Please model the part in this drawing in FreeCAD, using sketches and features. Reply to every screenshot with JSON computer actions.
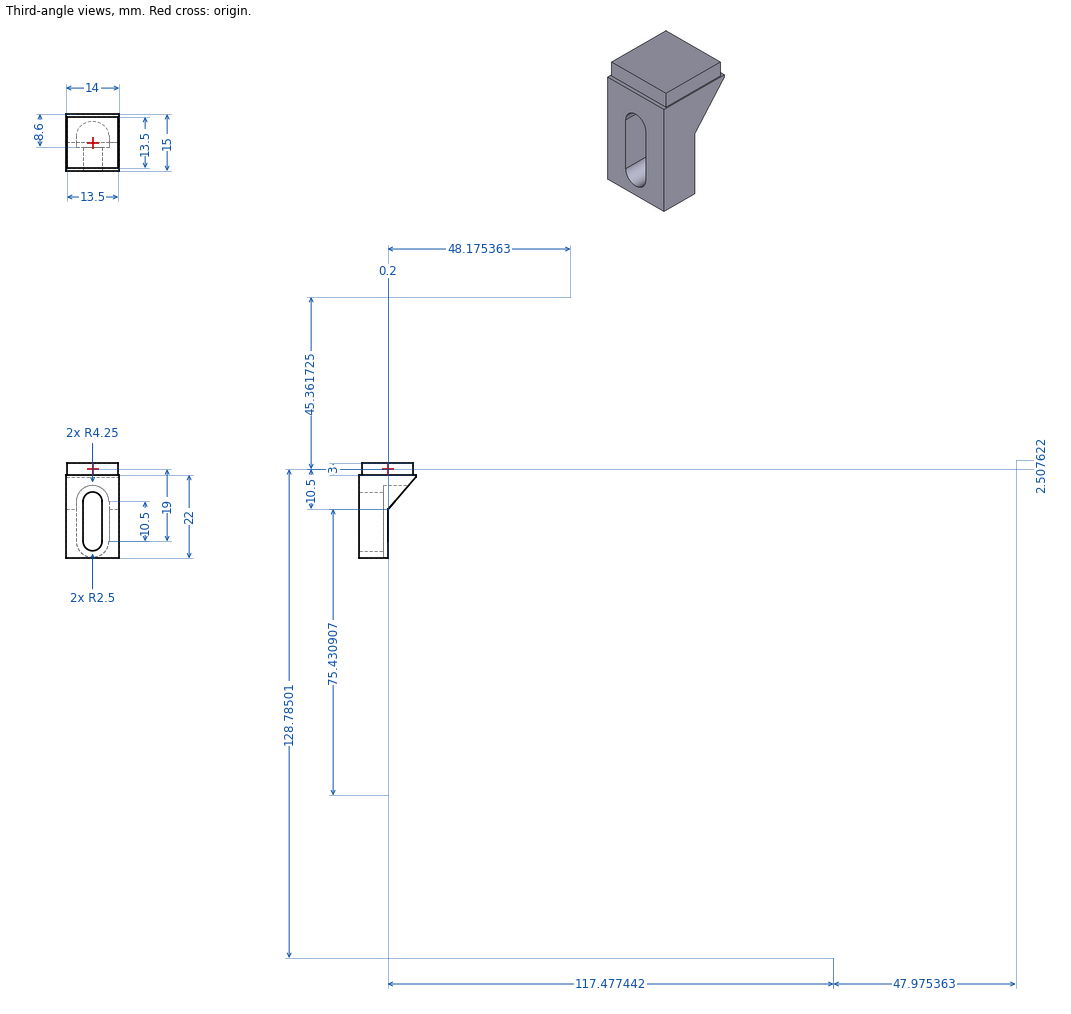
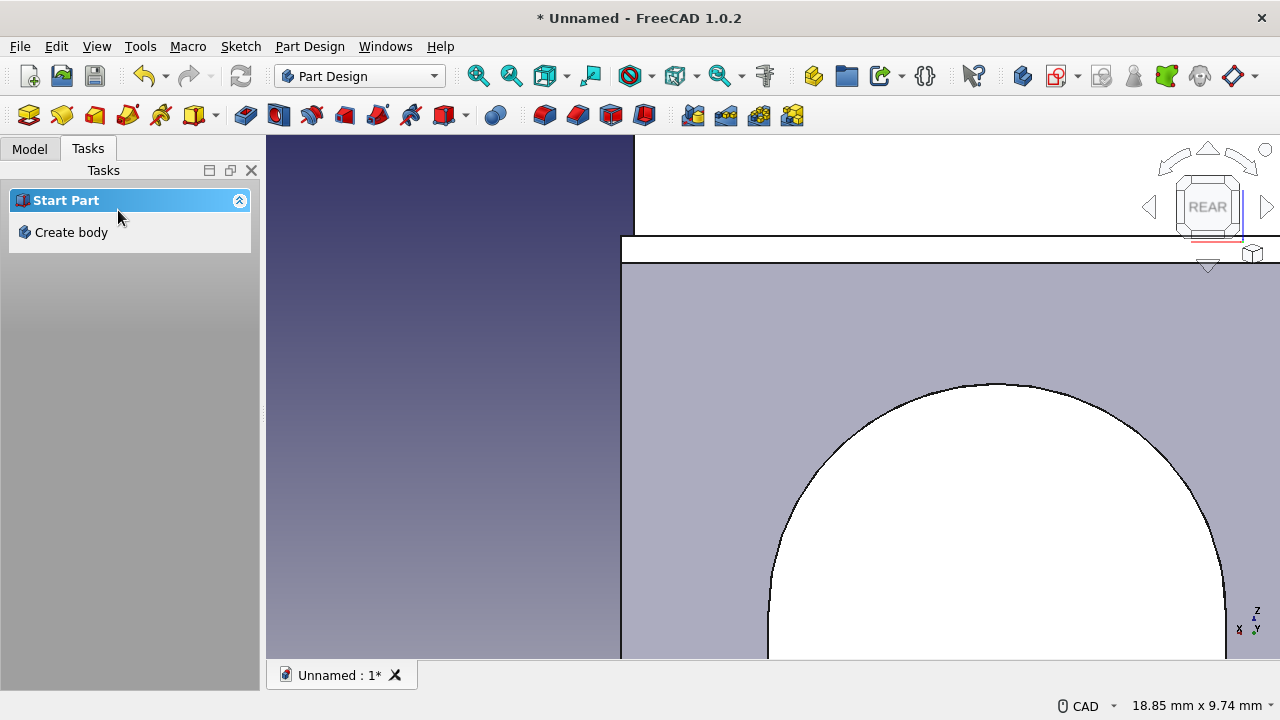
{"action": "key", "text": "v f"}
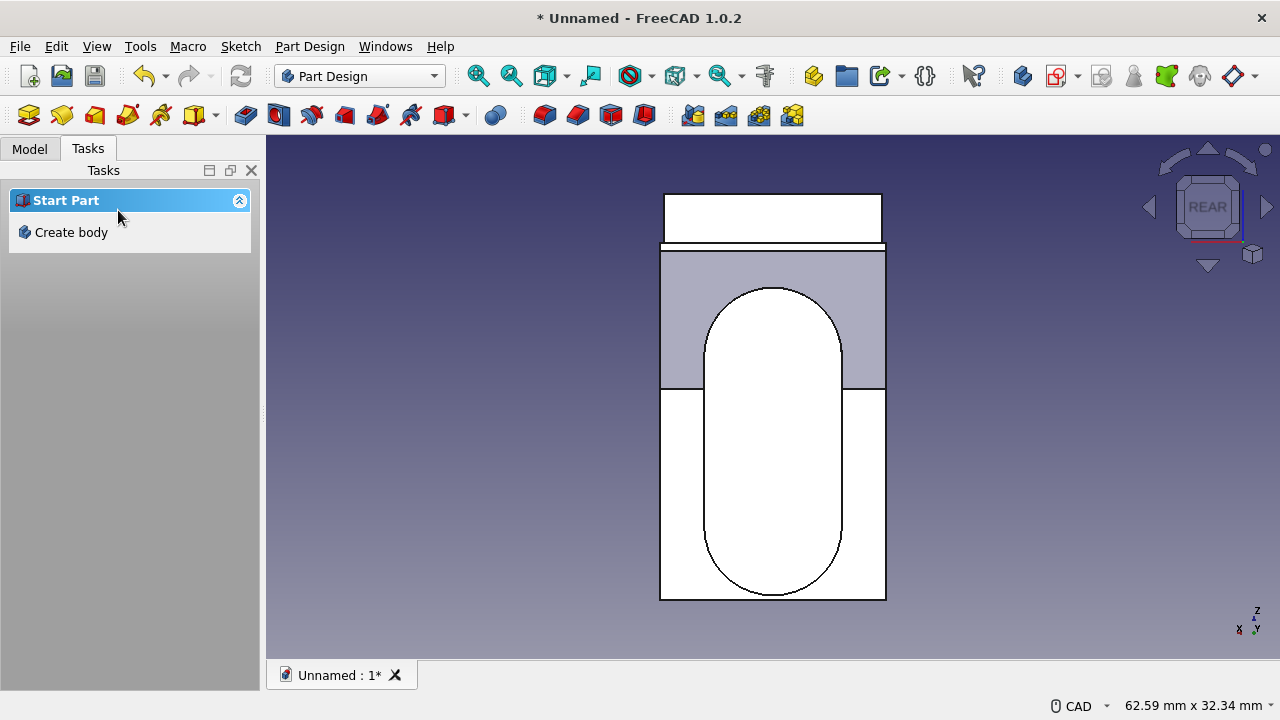
{"action": "left_click", "coordinate": [676, 433]}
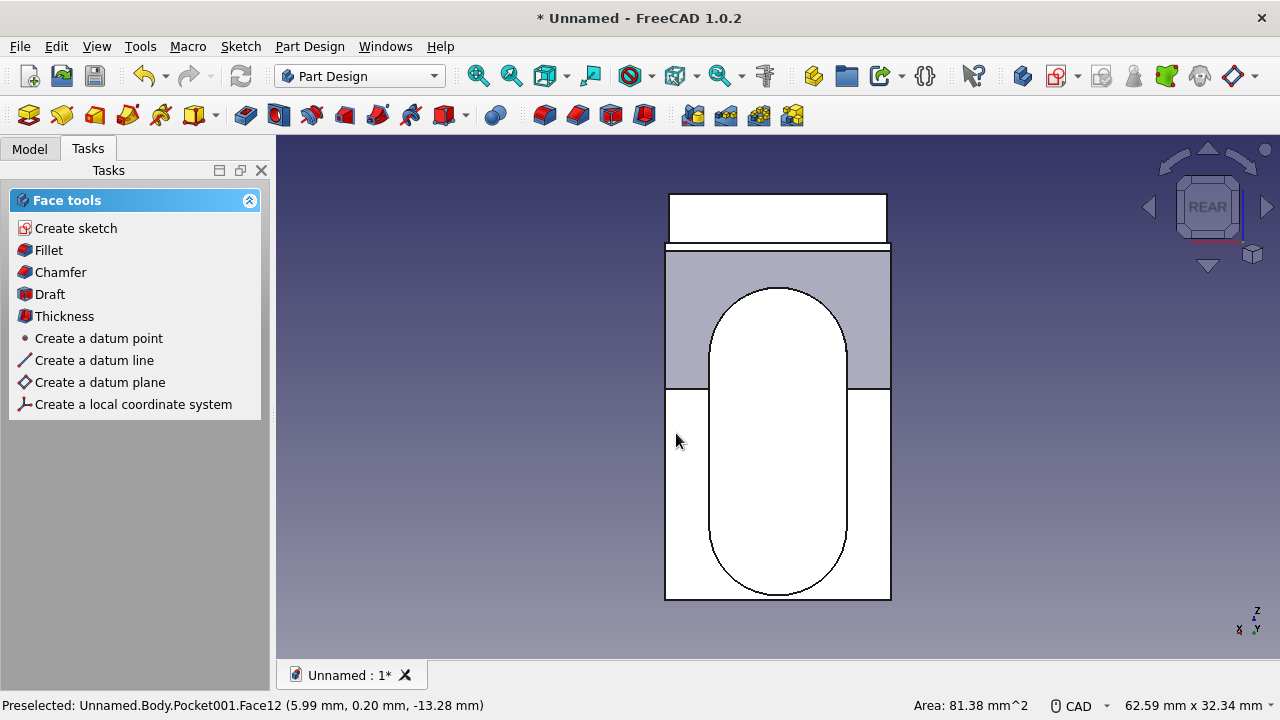
{"action": "left_click", "coordinate": [1056, 76]}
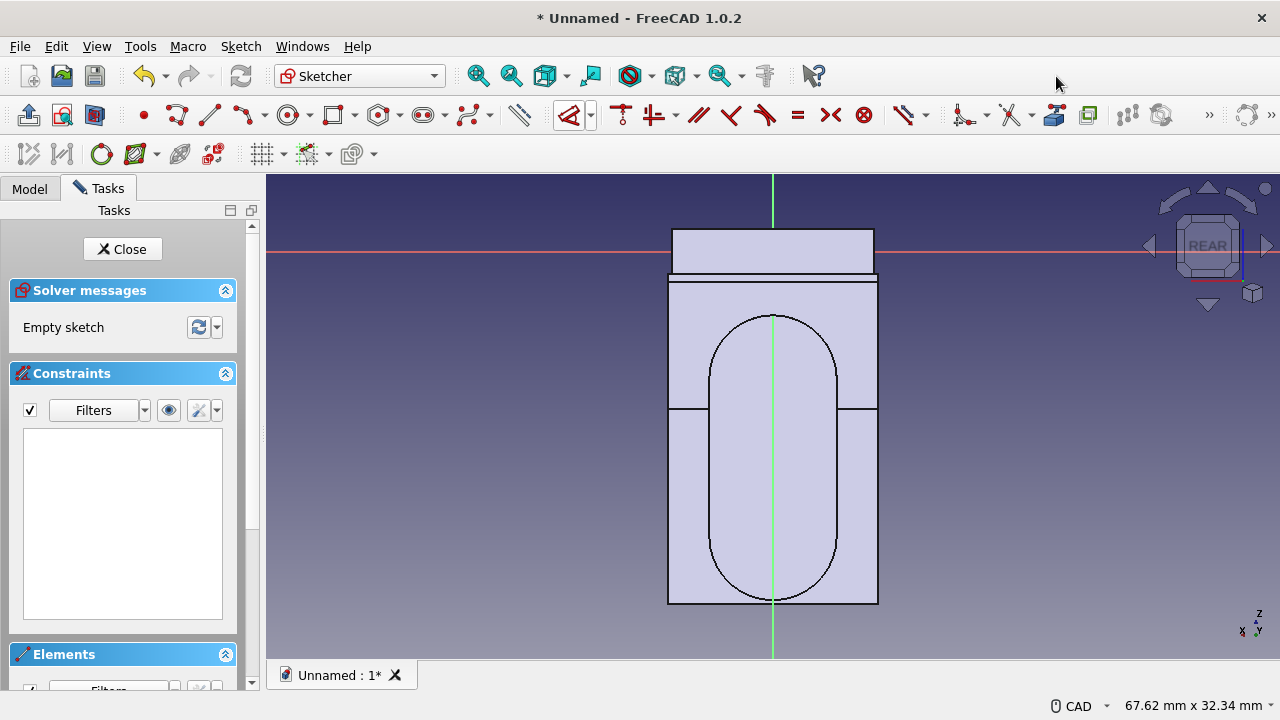
{"action": "key", "text": "g s"}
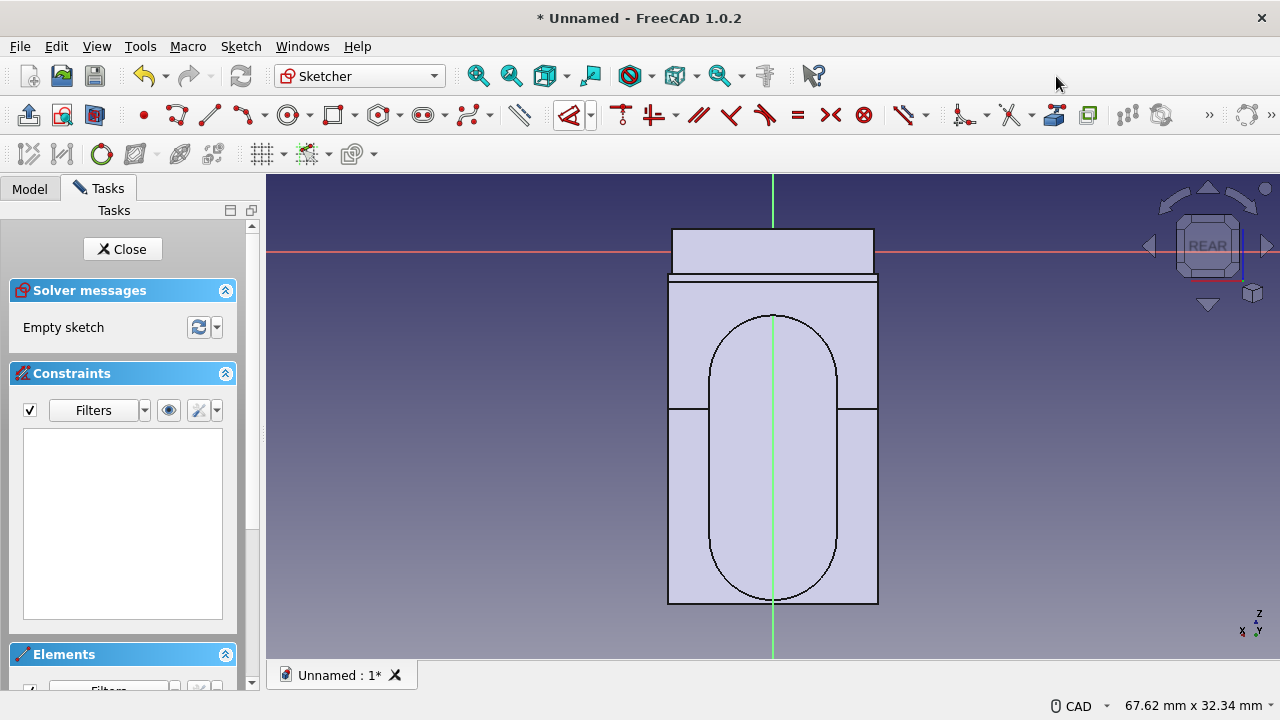
{"action": "left_click", "coordinate": [773, 536]}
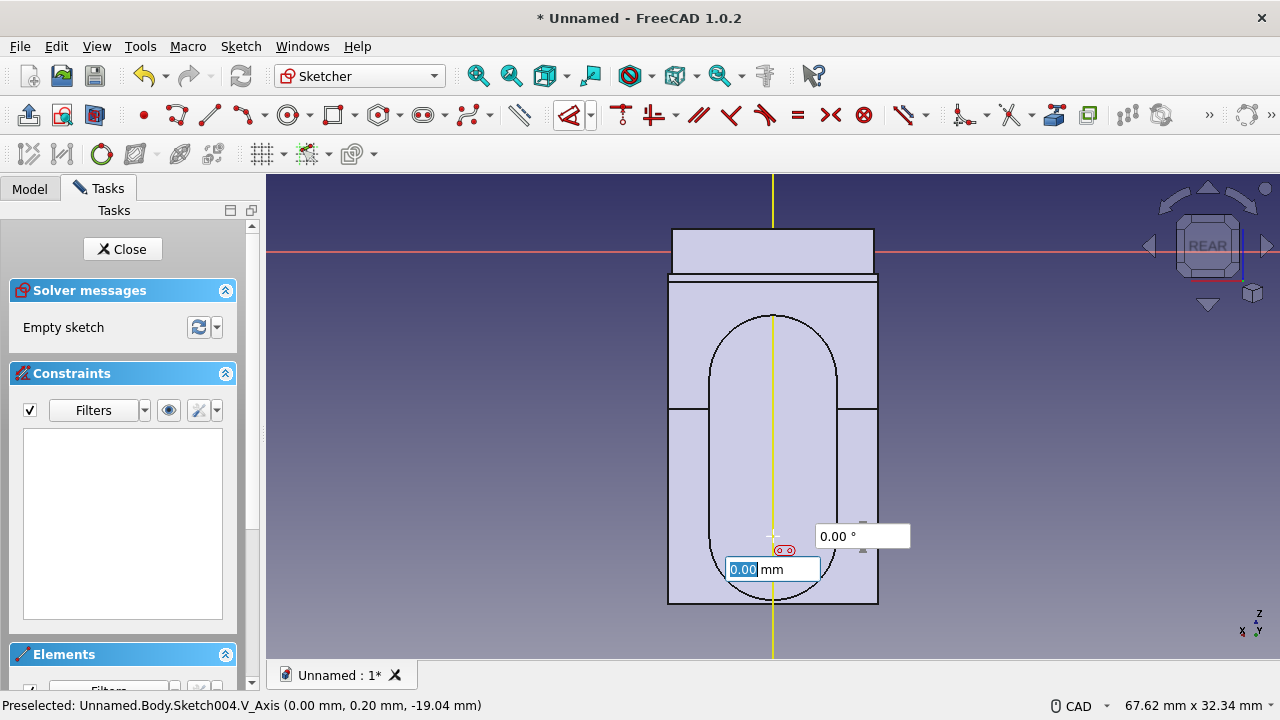
{"action": "left_click", "coordinate": [782, 379]}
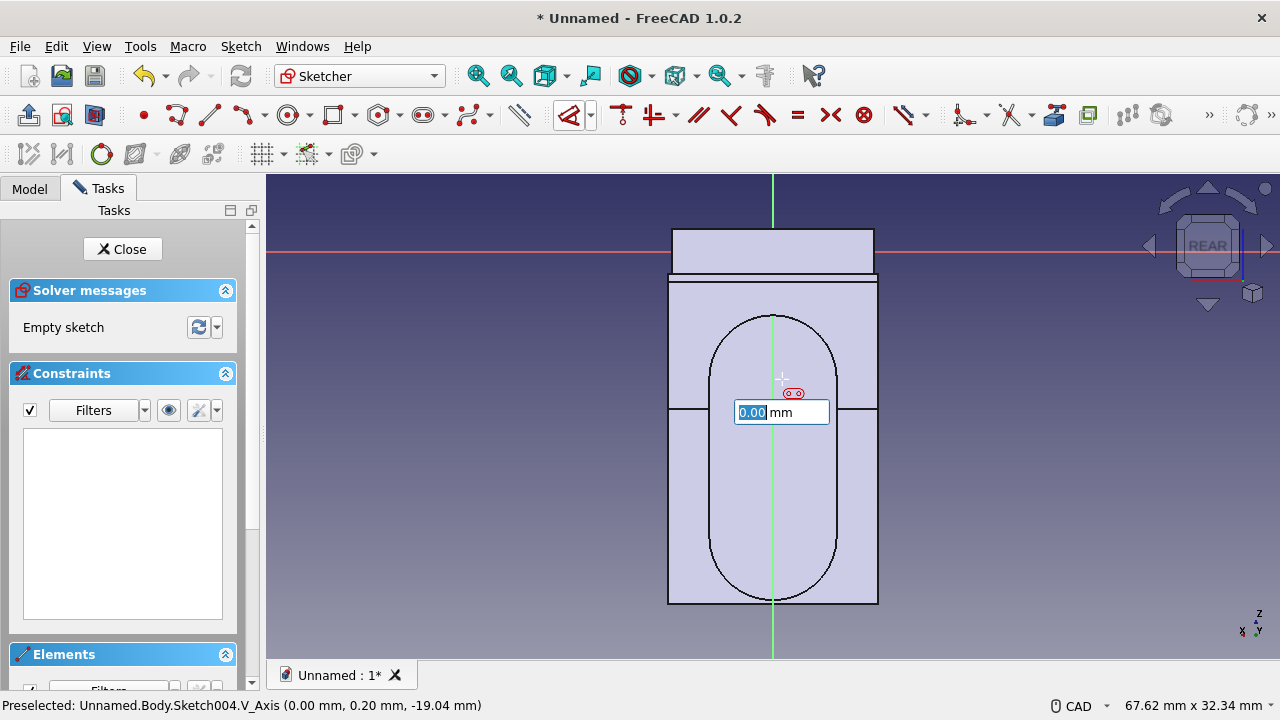
{"action": "left_click", "coordinate": [736, 458]}
{"action": "key", "text": "Escape"}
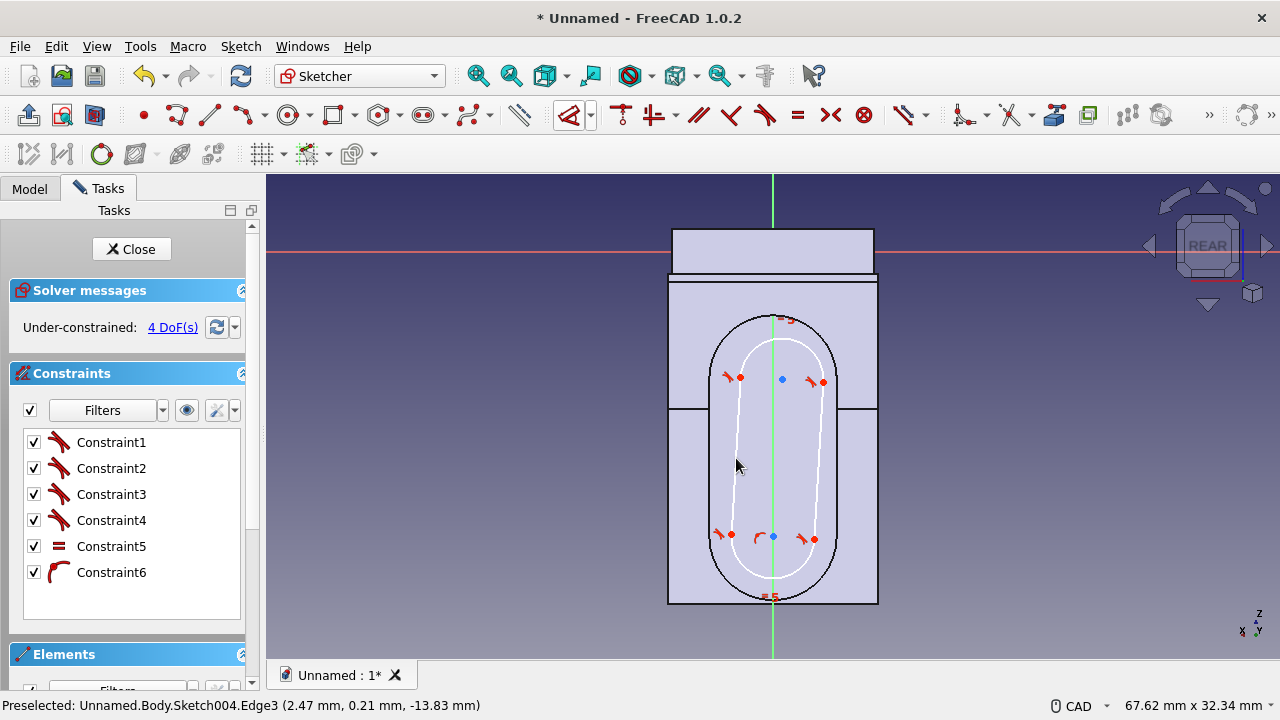
{"action": "left_click", "coordinate": [734, 488]}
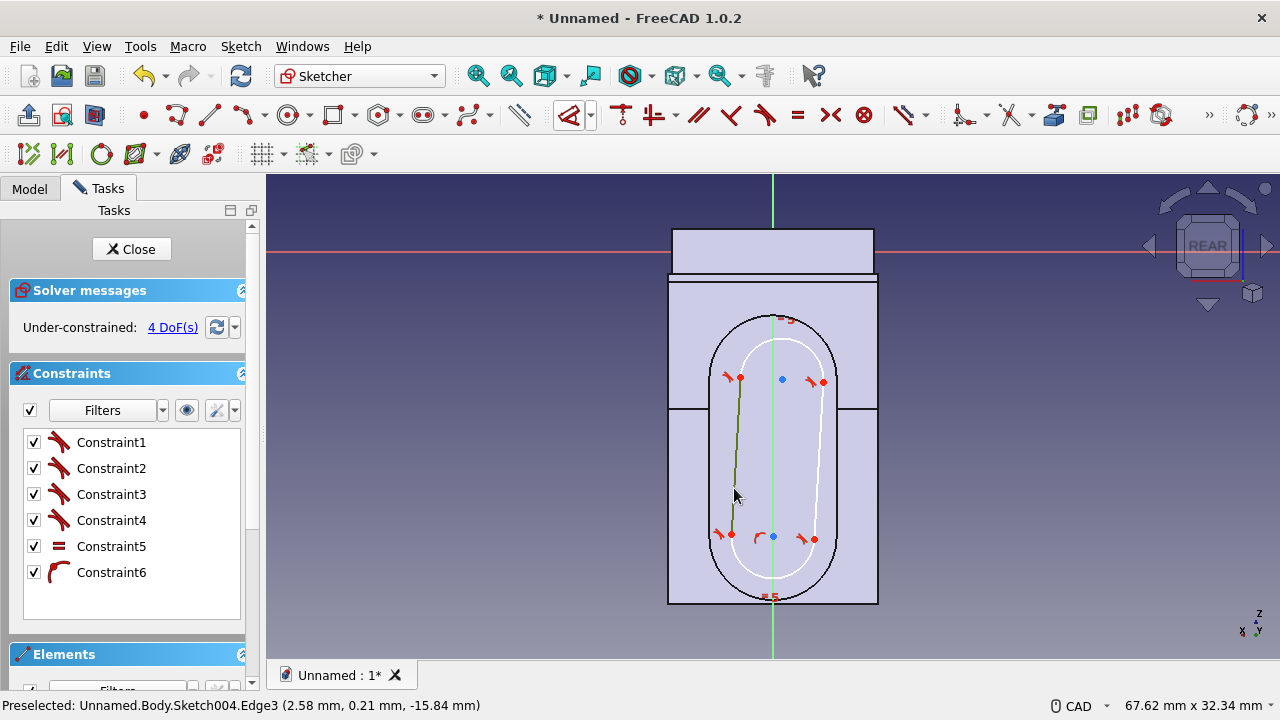
{"action": "key", "text": "v"}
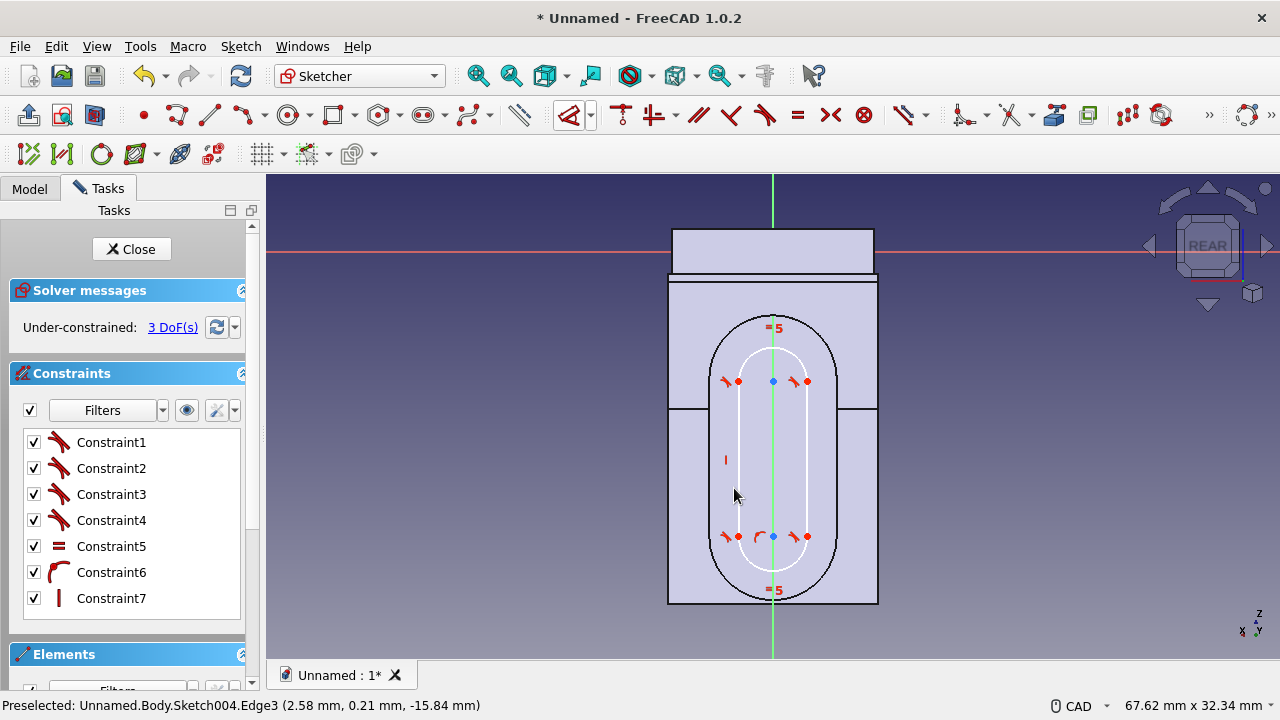
{"action": "left_click", "coordinate": [753, 565]}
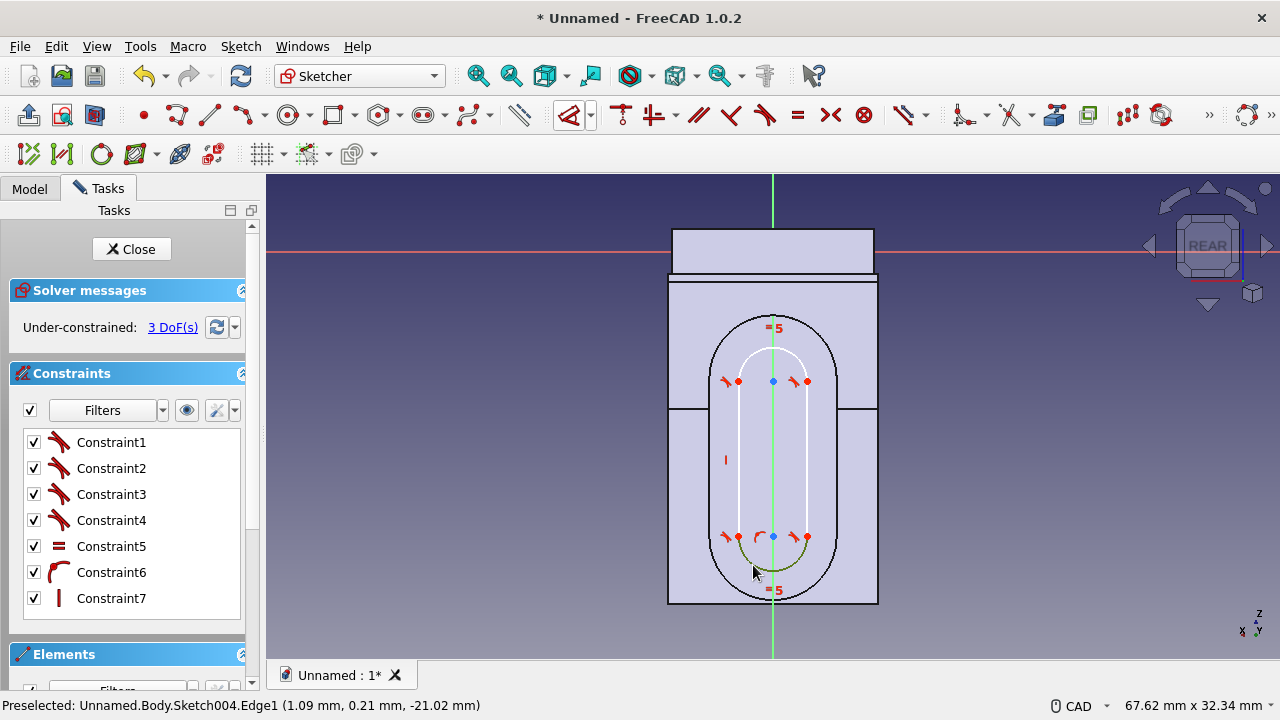
{"action": "key", "text": "k r"}